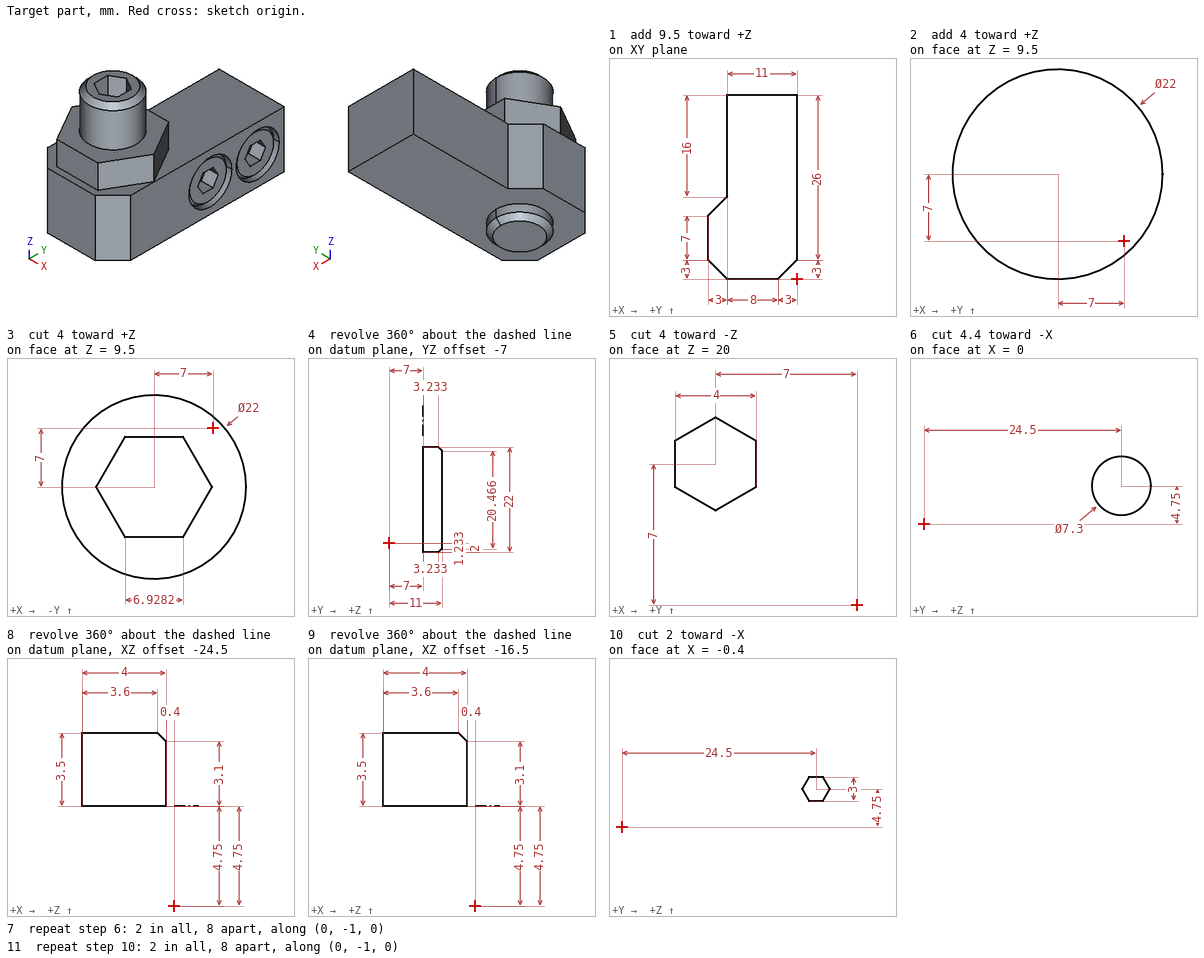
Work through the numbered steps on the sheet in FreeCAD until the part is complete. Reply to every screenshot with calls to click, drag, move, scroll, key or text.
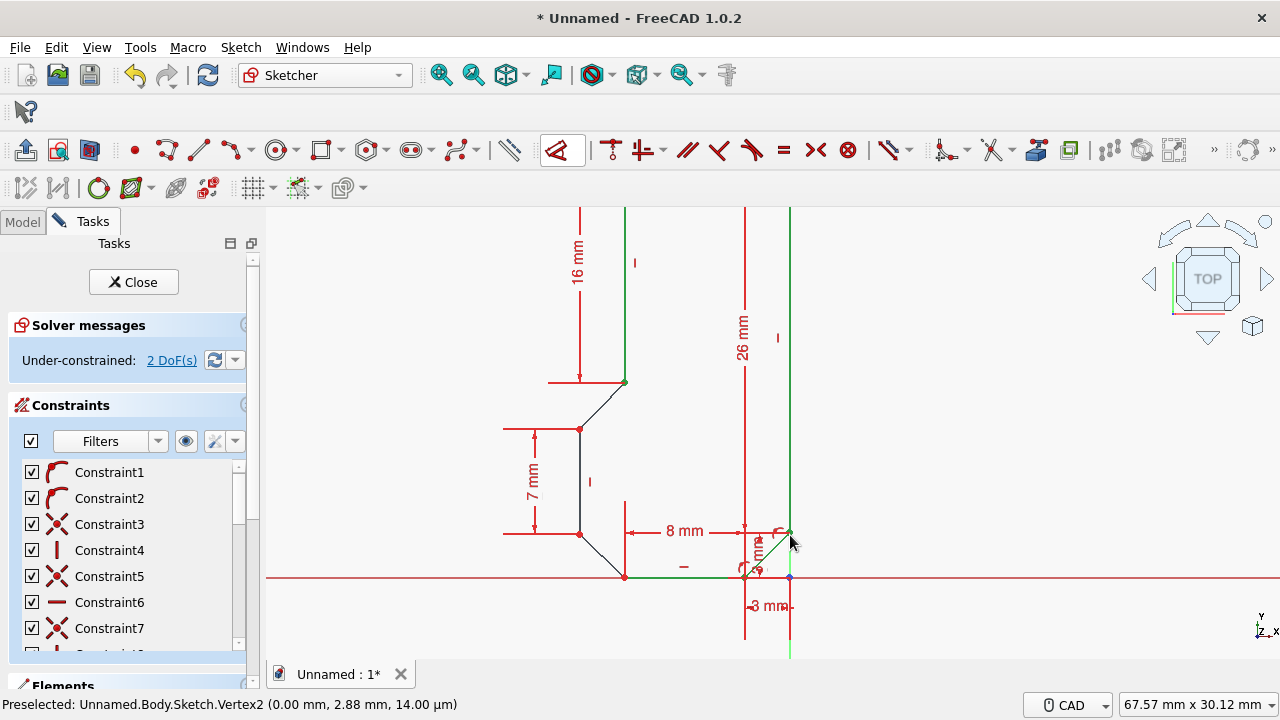
click(580, 534)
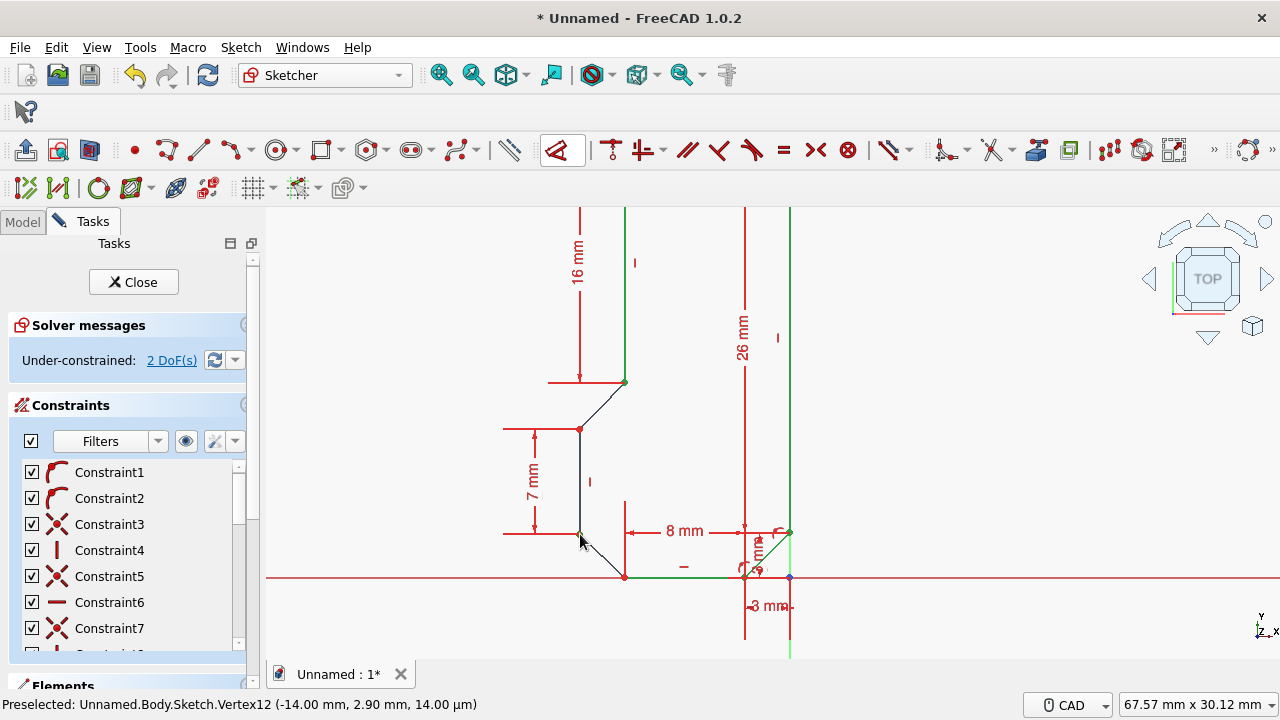
key(i)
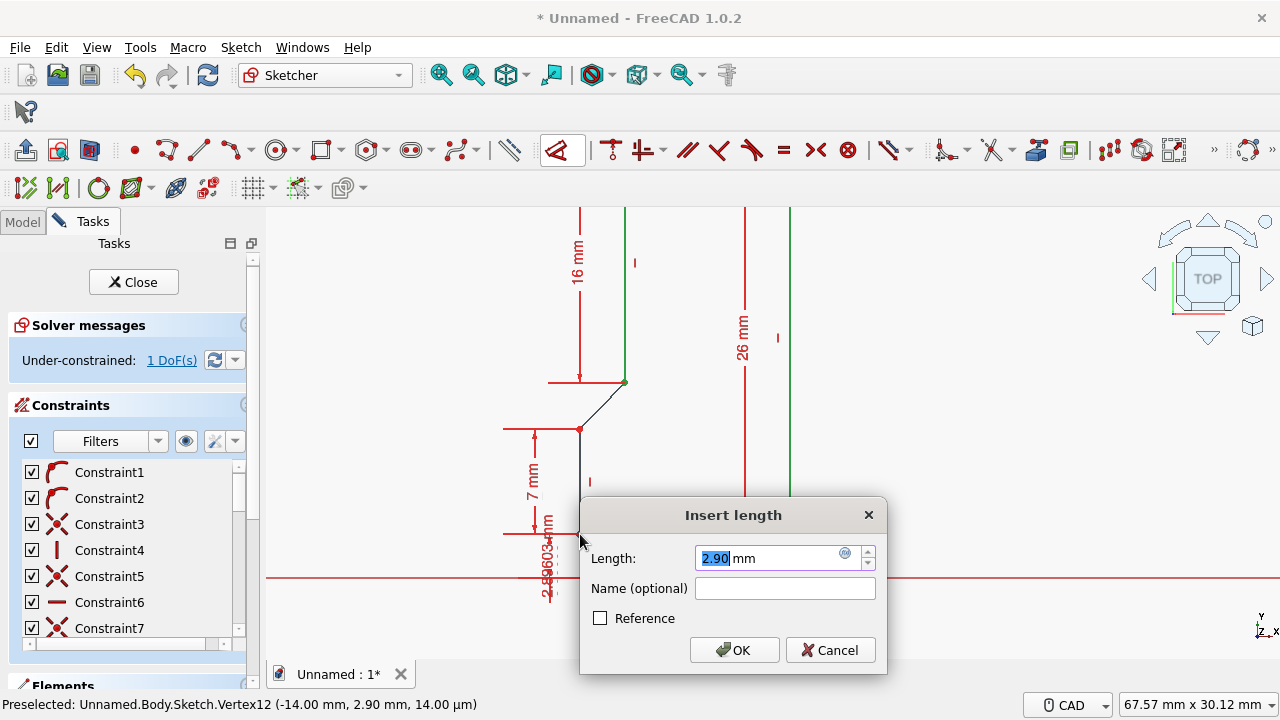
text(3)
key(Return)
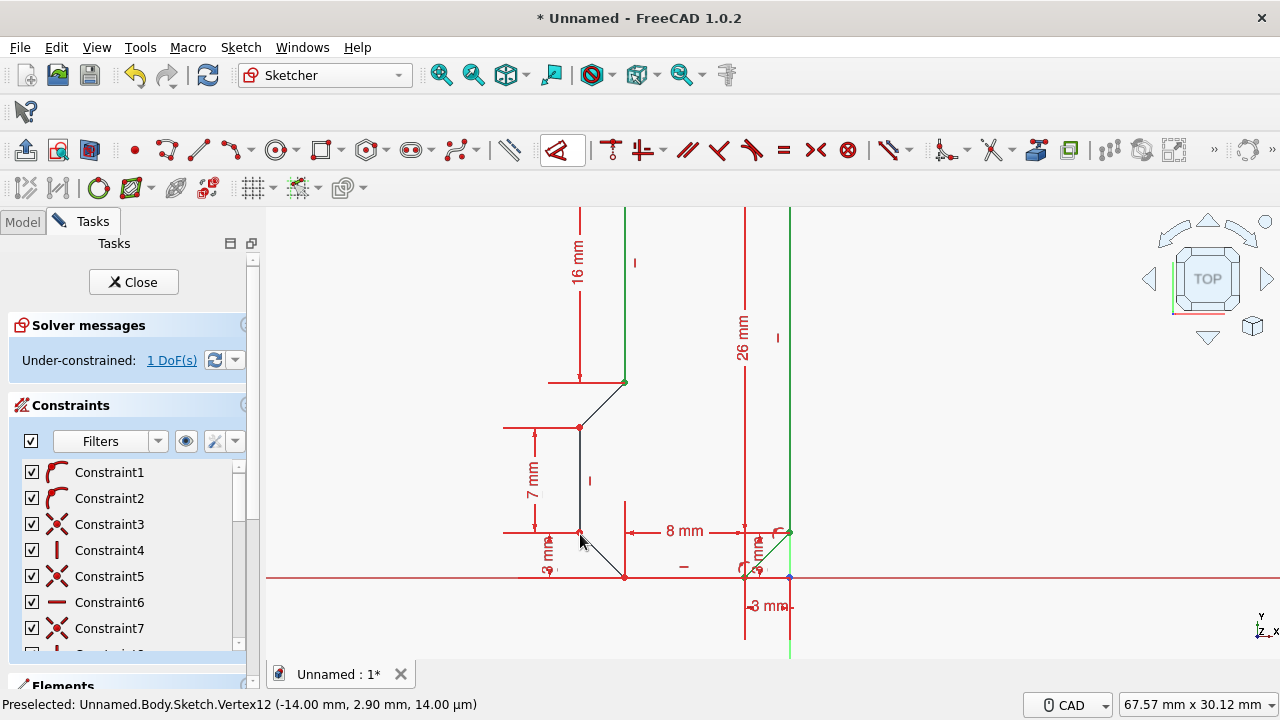
click(611, 396)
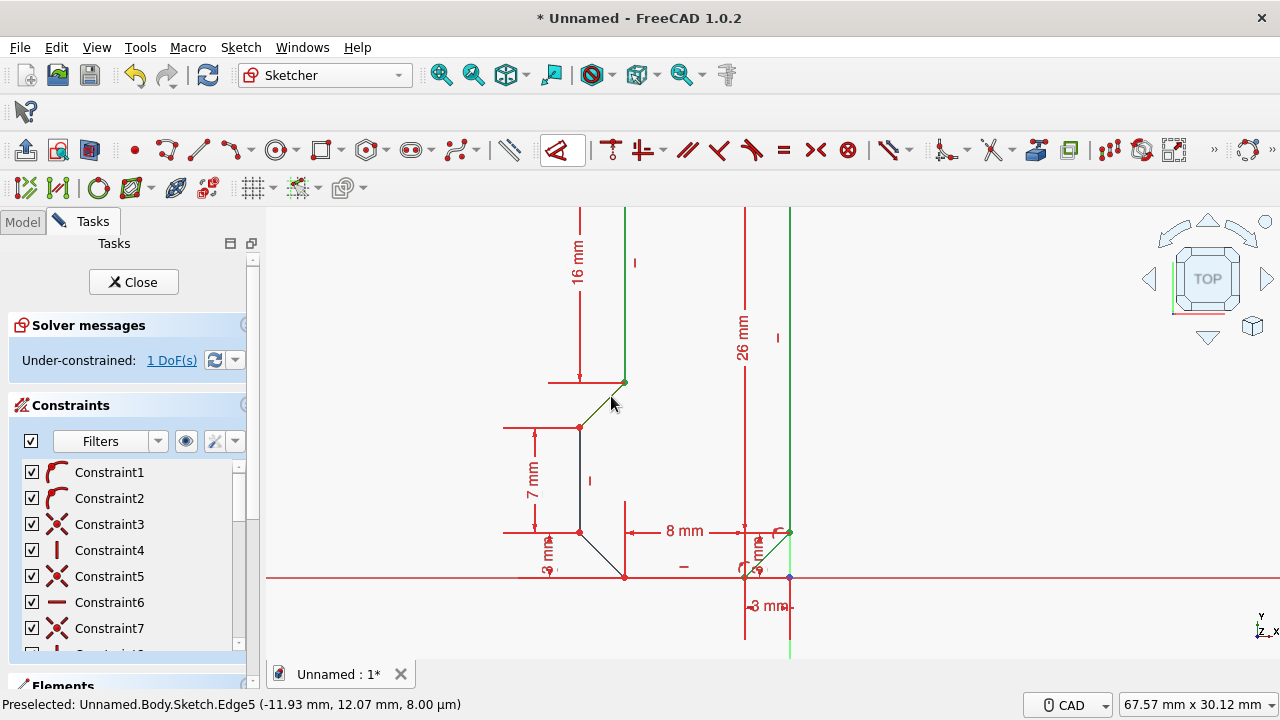
key(l)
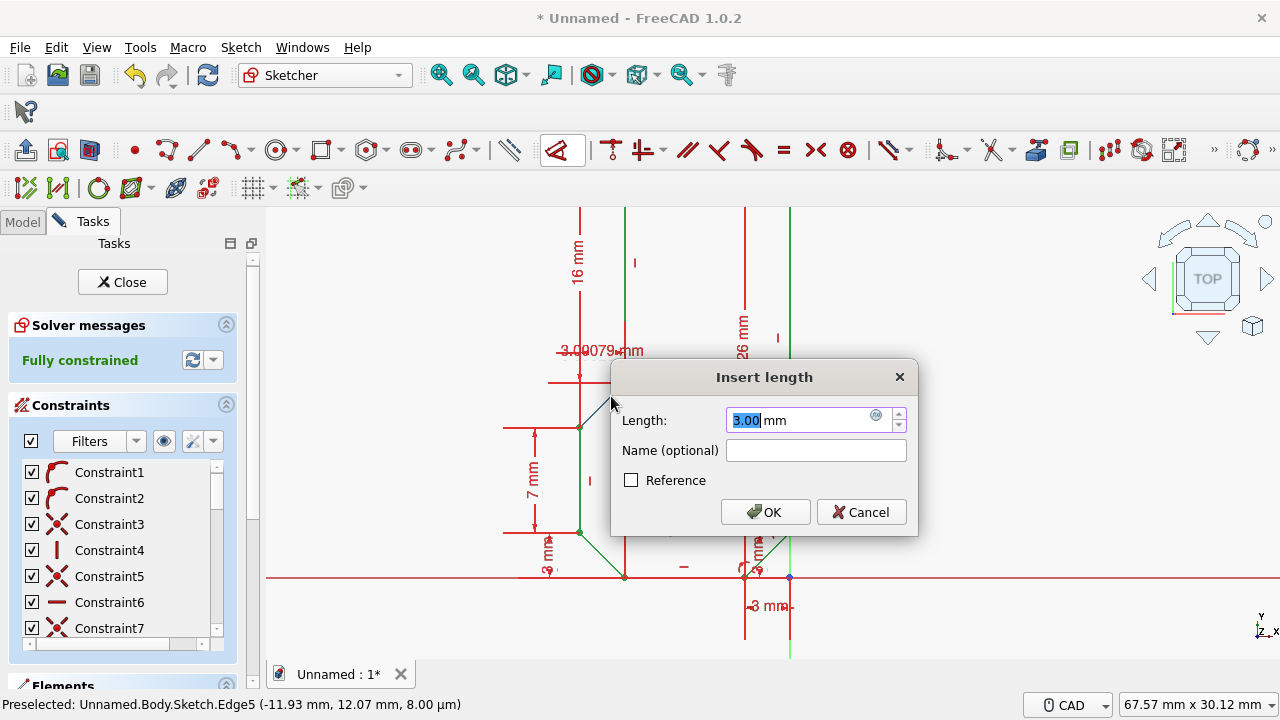
text(3)
key(Return)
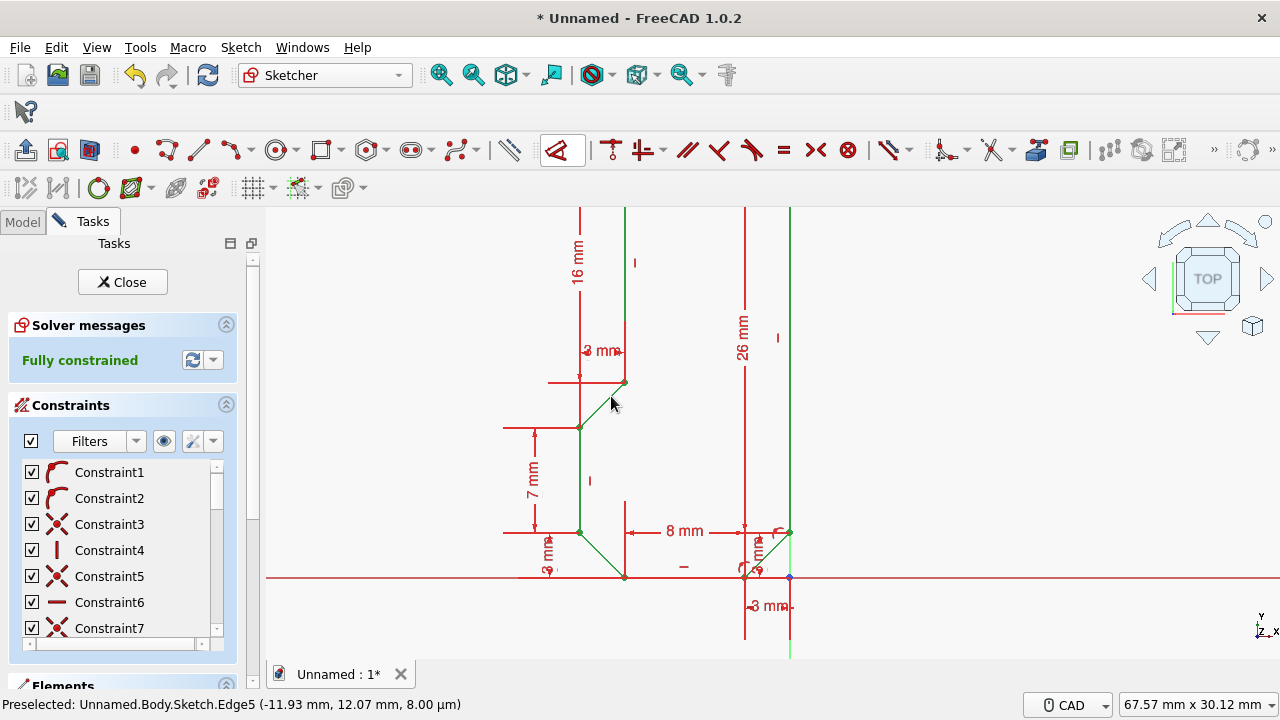
click(123, 282)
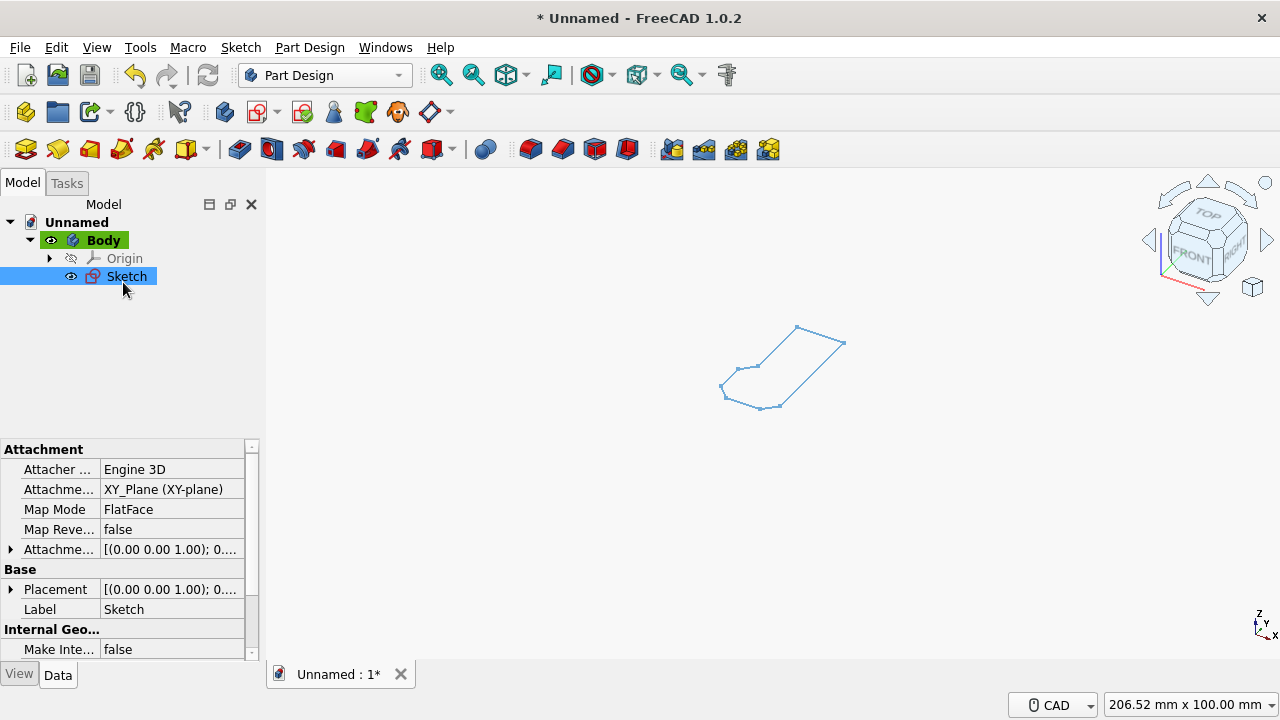
click(26, 150)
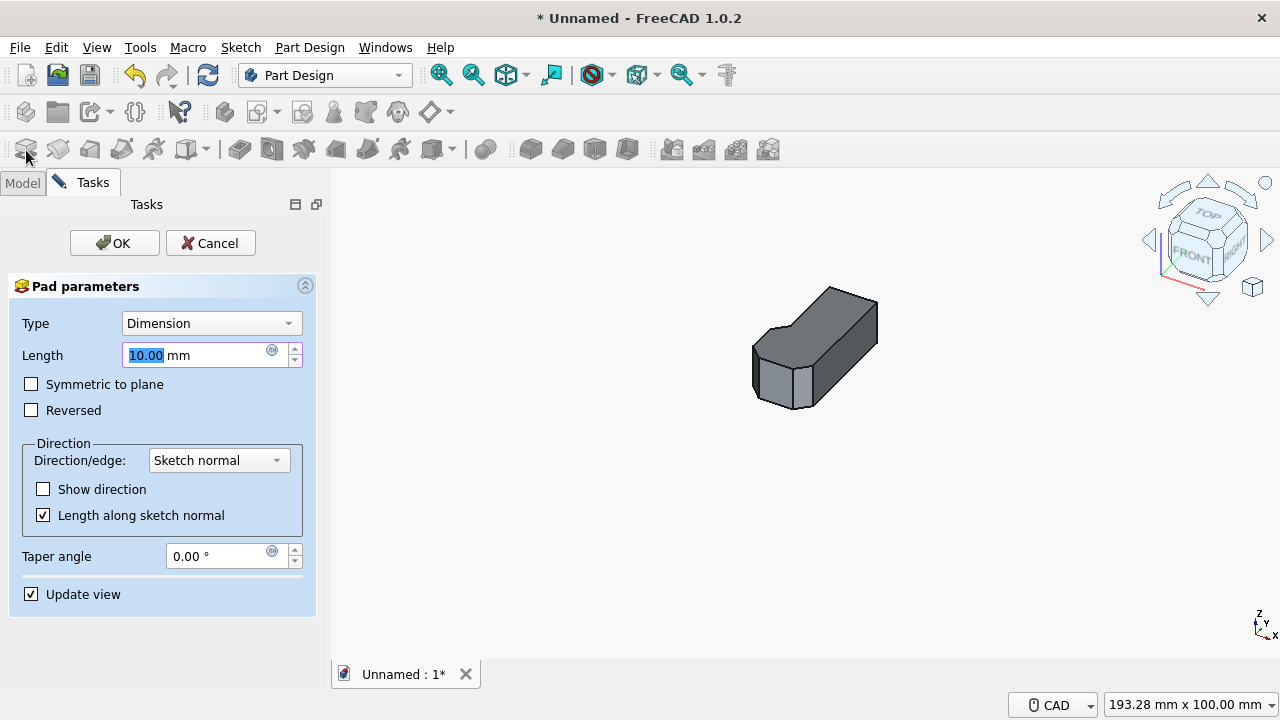
text(9.5)
key(Tab)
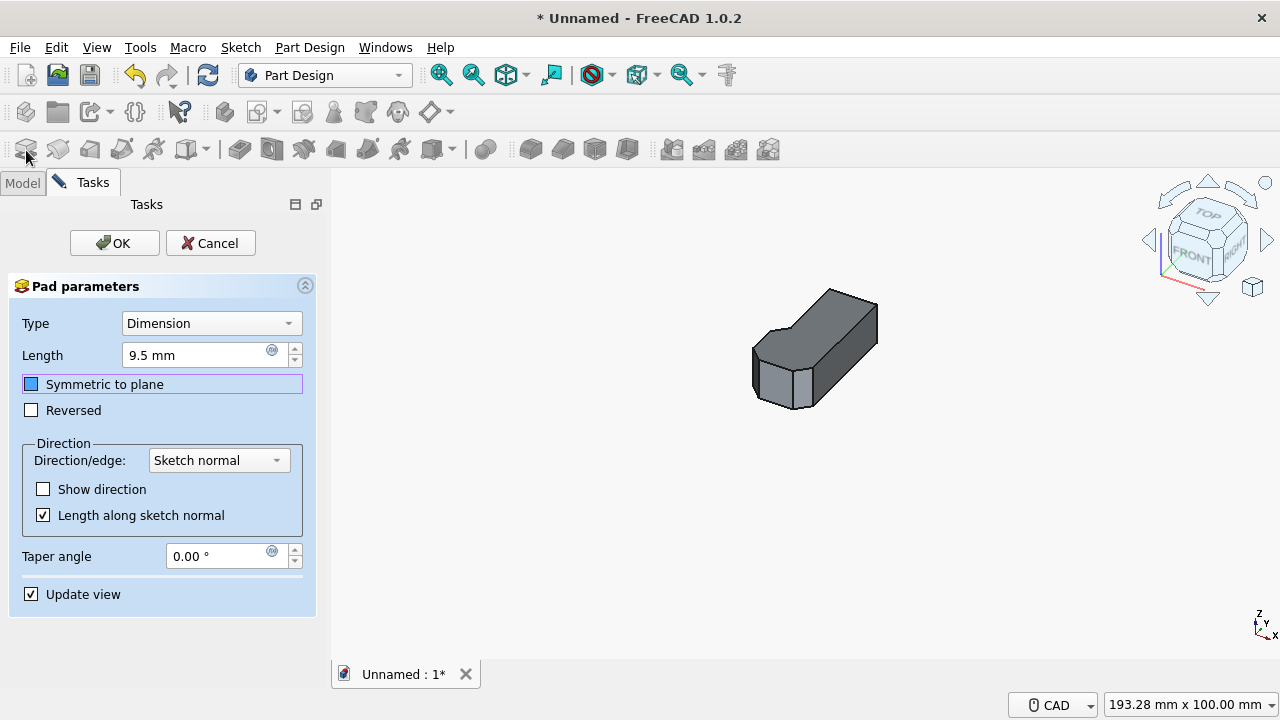
click(115, 243)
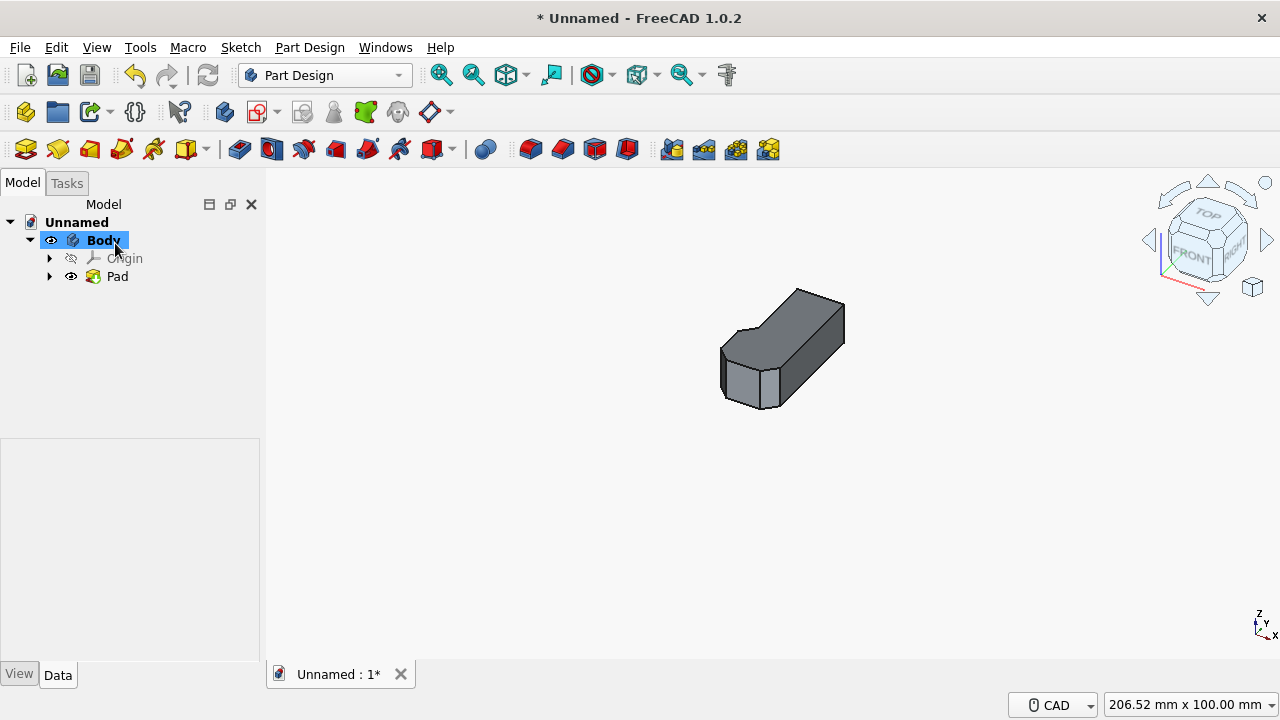
key(v)
key(f)